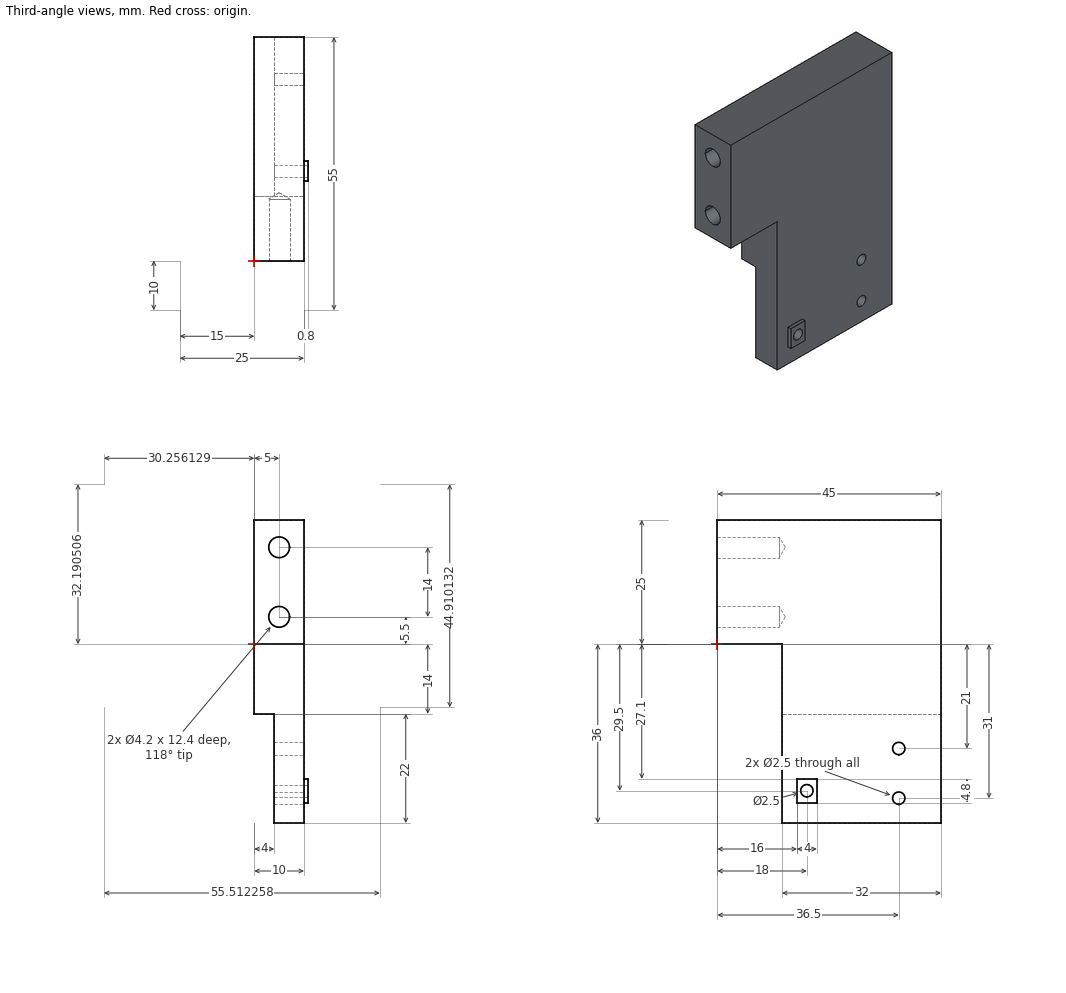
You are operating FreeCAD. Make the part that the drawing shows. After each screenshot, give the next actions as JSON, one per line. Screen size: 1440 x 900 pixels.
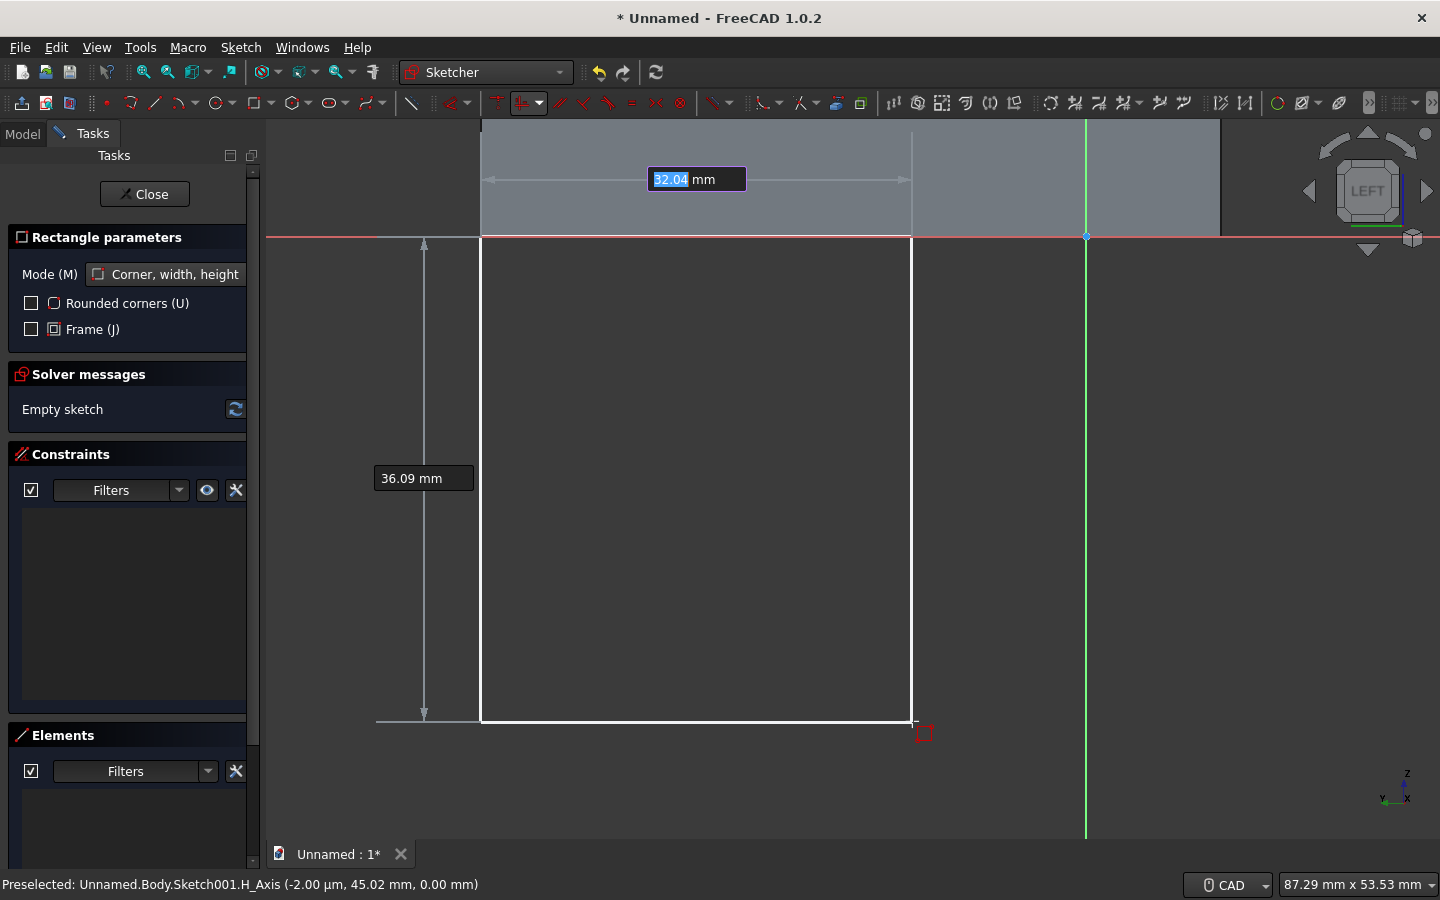
{"action": "type", "text": "32"}
{"action": "key", "text": "Tab"}
{"action": "type", "text": "36"}
{"action": "key", "text": "Return"}
{"action": "key", "text": "Escape"}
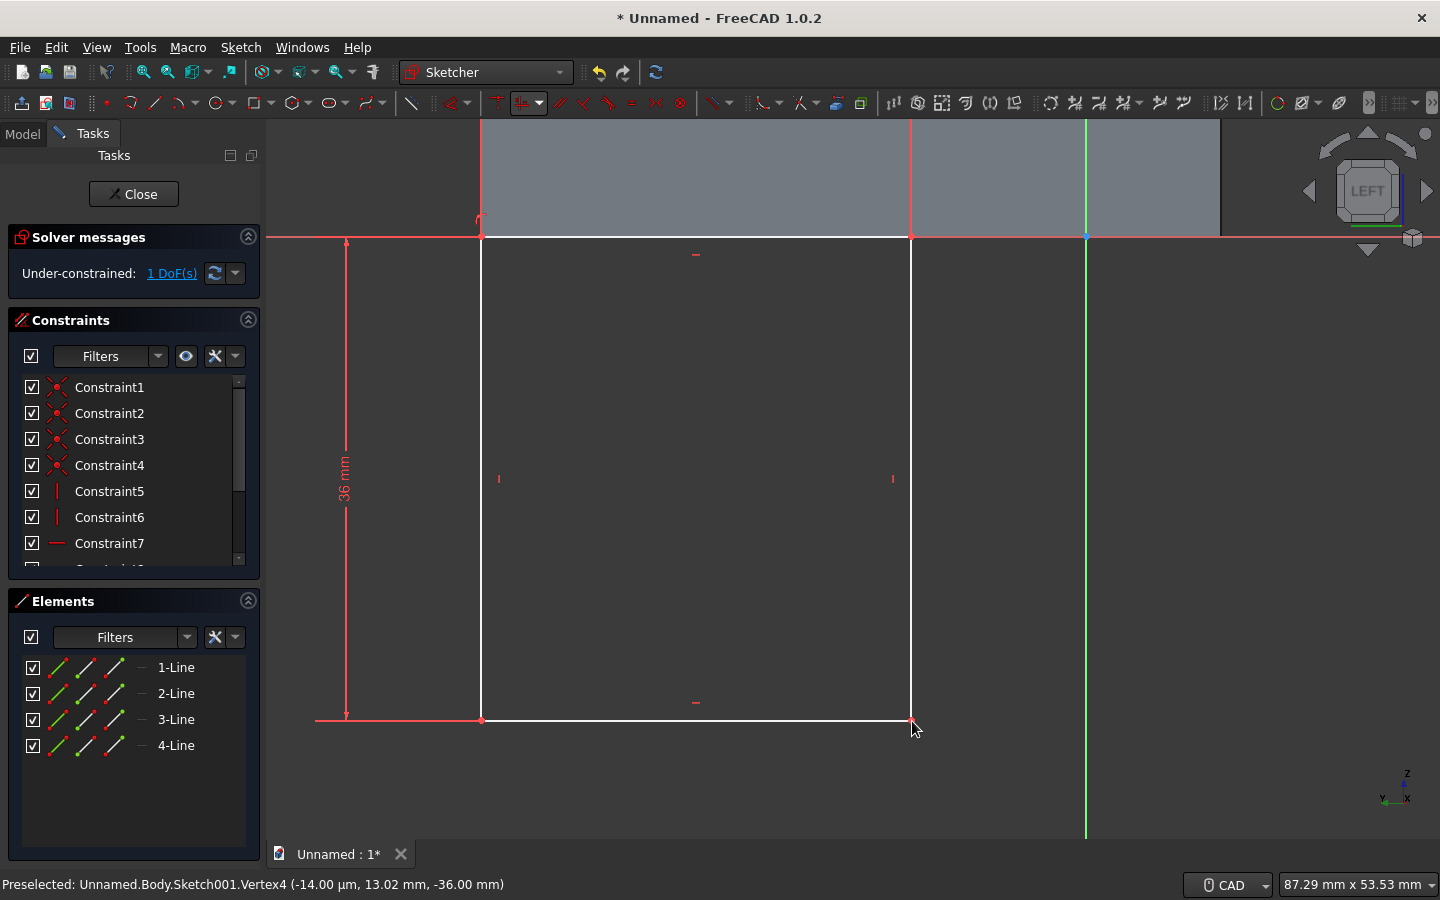
{"action": "left_click", "coordinate": [481, 237]}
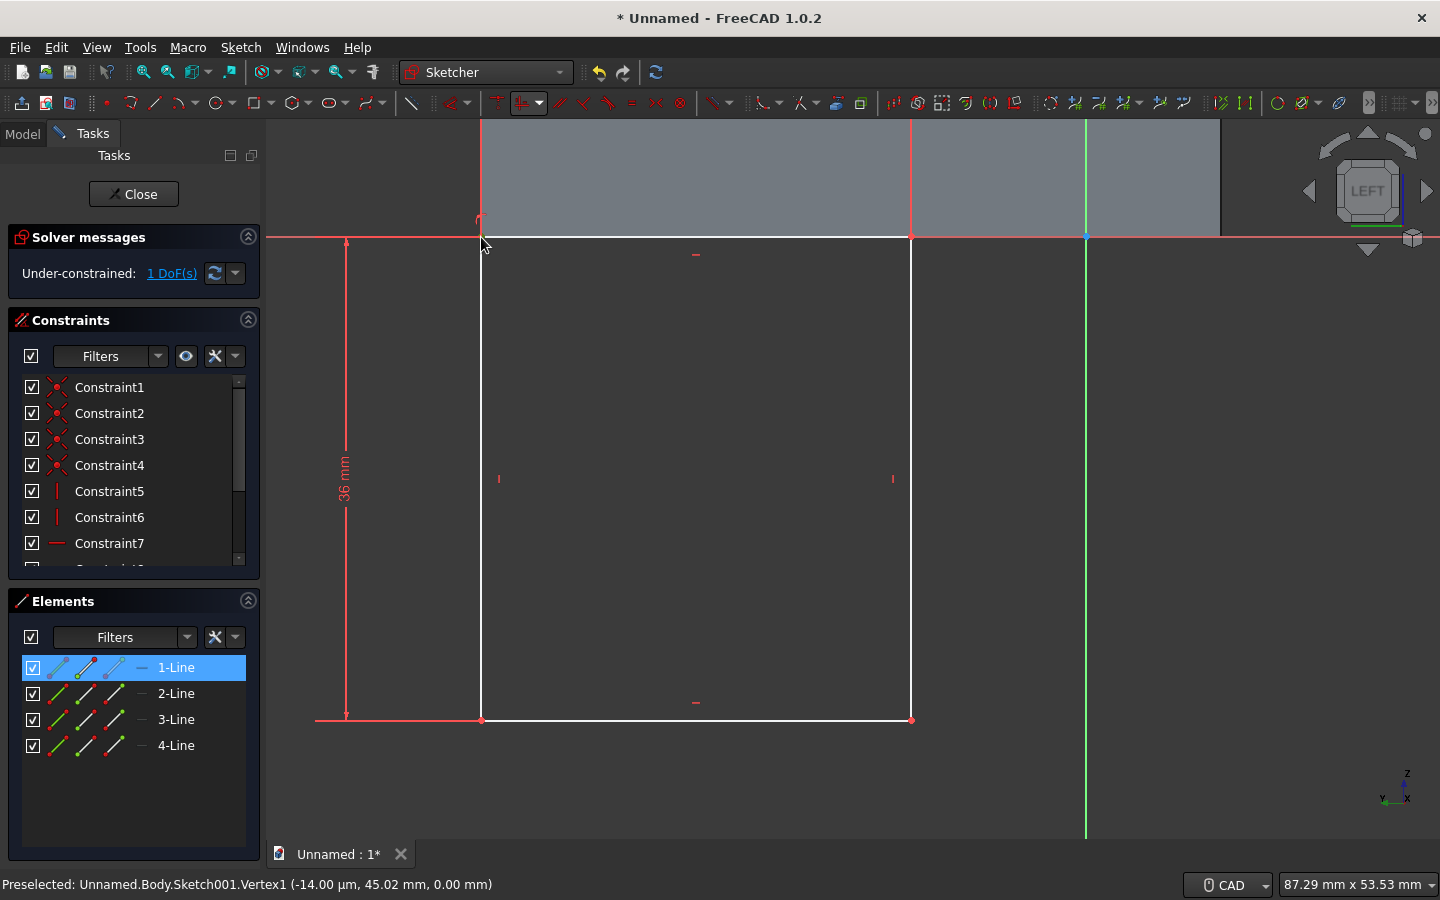
{"action": "left_click", "coordinate": [470, 104]}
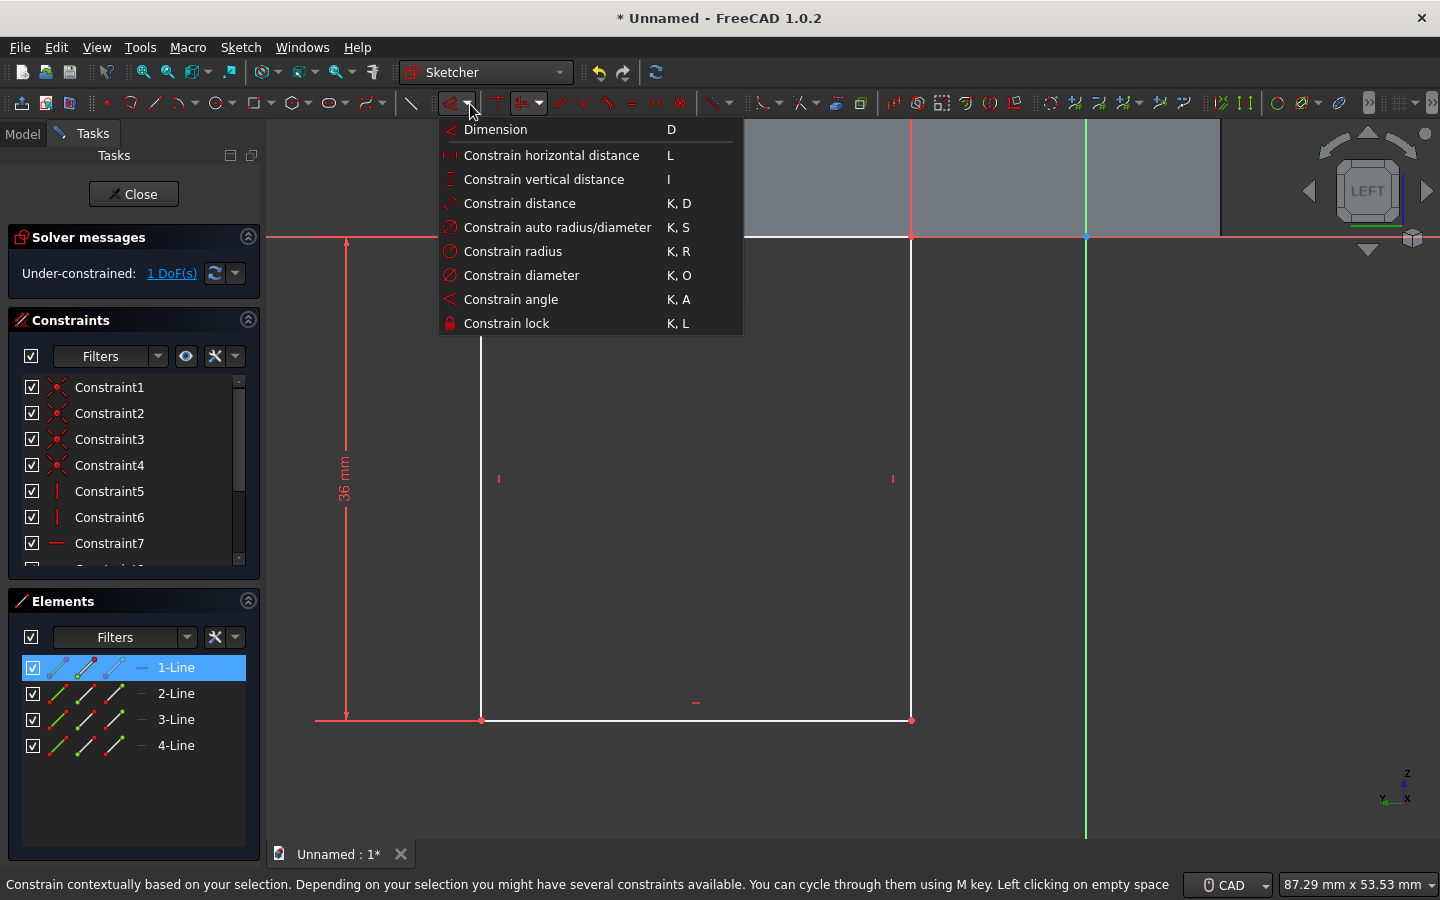
{"action": "left_click", "coordinate": [591, 155]}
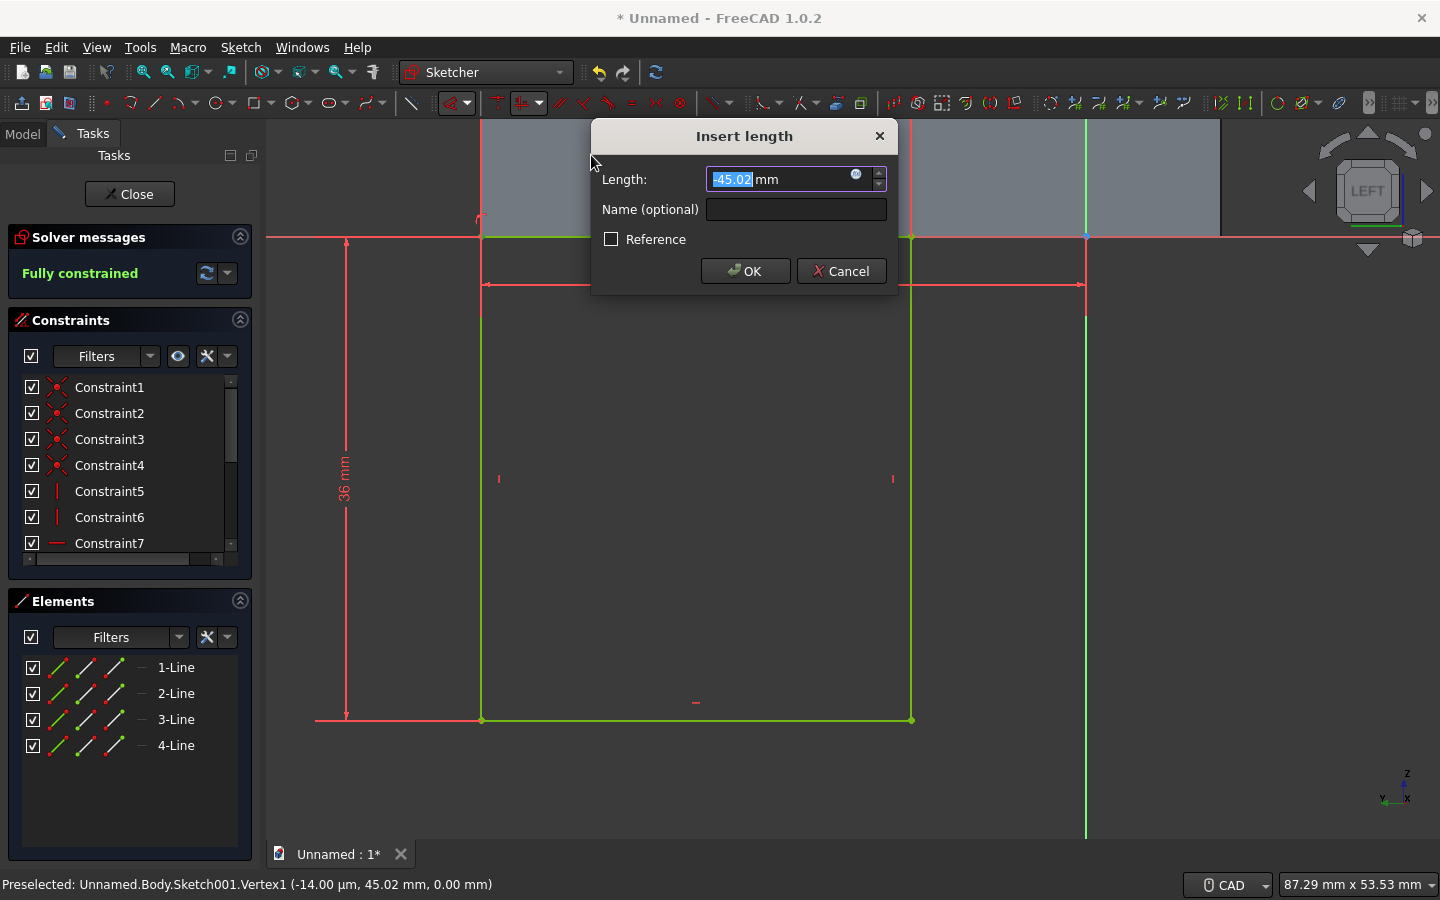
{"action": "type", "text": "-45"}
{"action": "key", "text": "Return"}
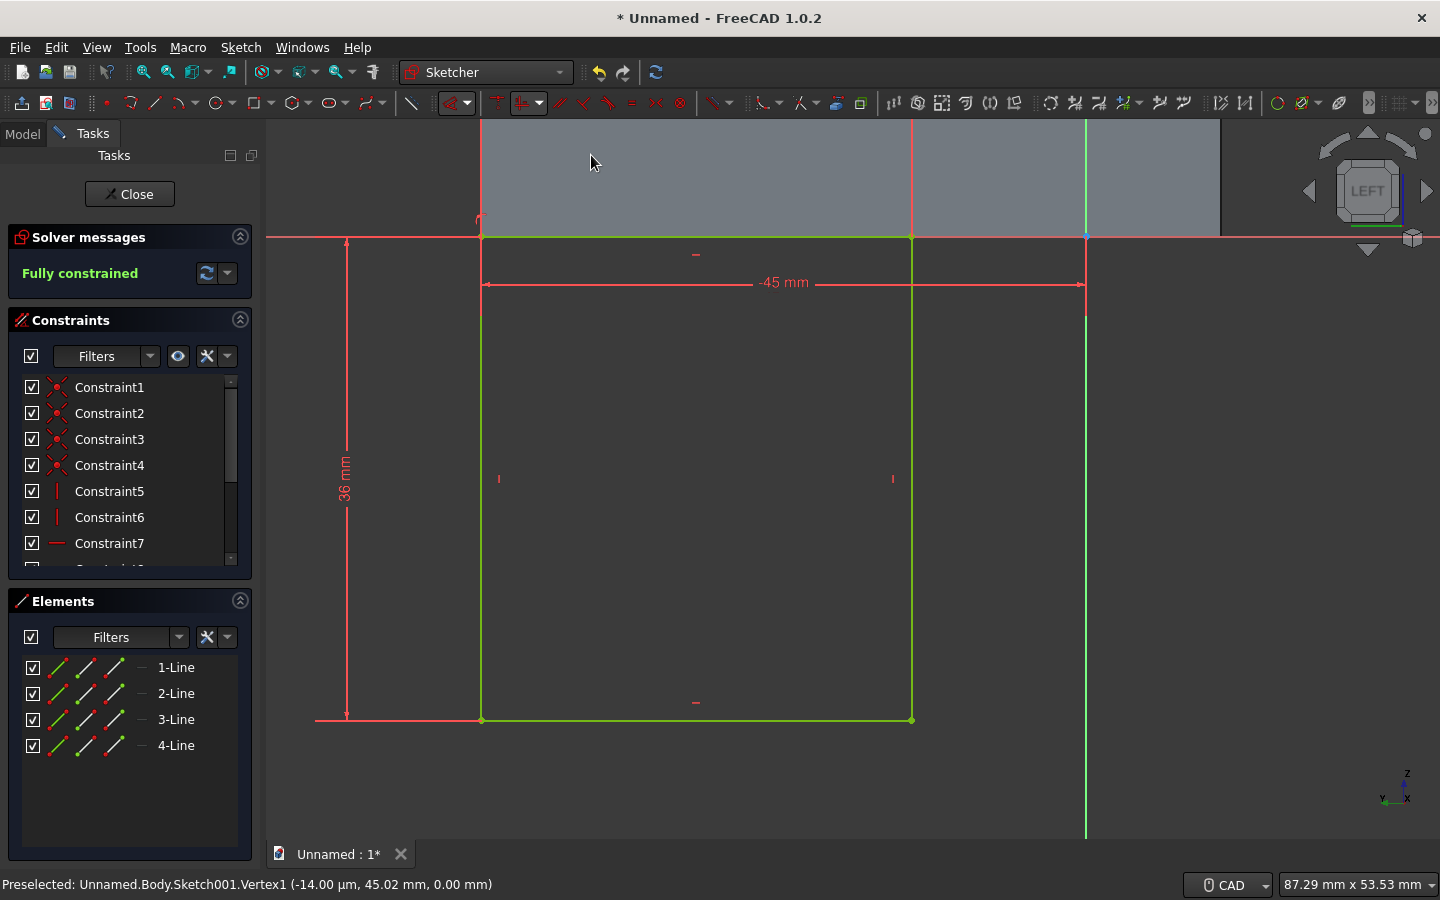
{"action": "left_click", "coordinate": [130, 194]}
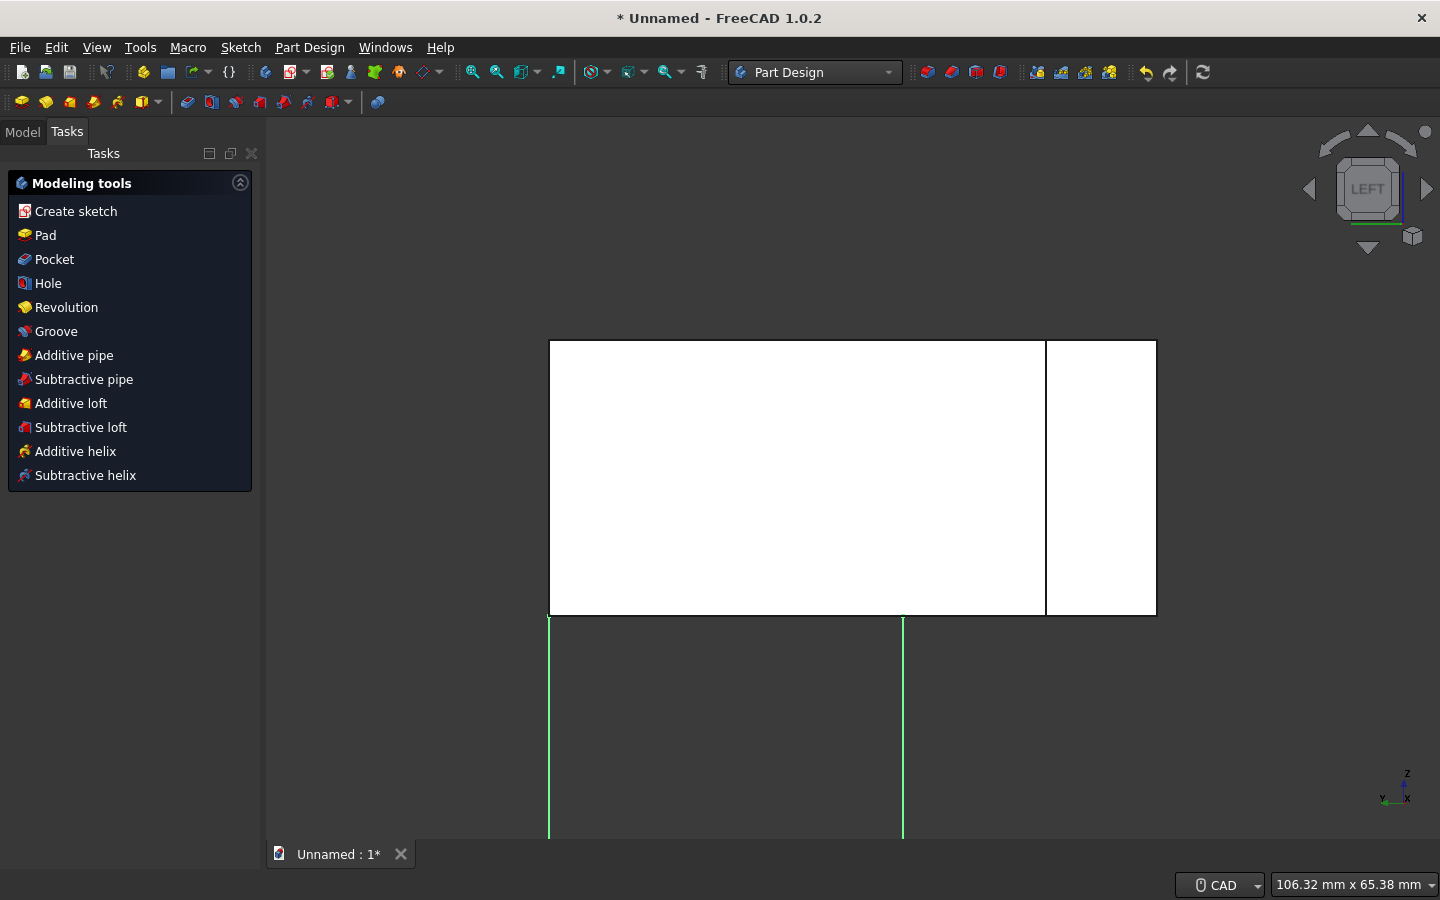
{"action": "left_click", "coordinate": [22, 102]}